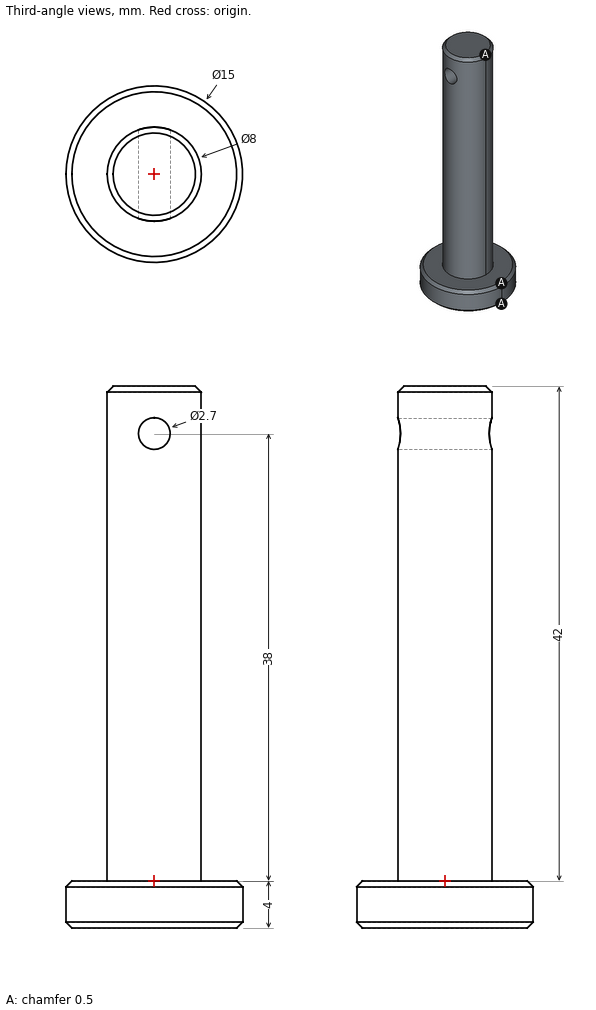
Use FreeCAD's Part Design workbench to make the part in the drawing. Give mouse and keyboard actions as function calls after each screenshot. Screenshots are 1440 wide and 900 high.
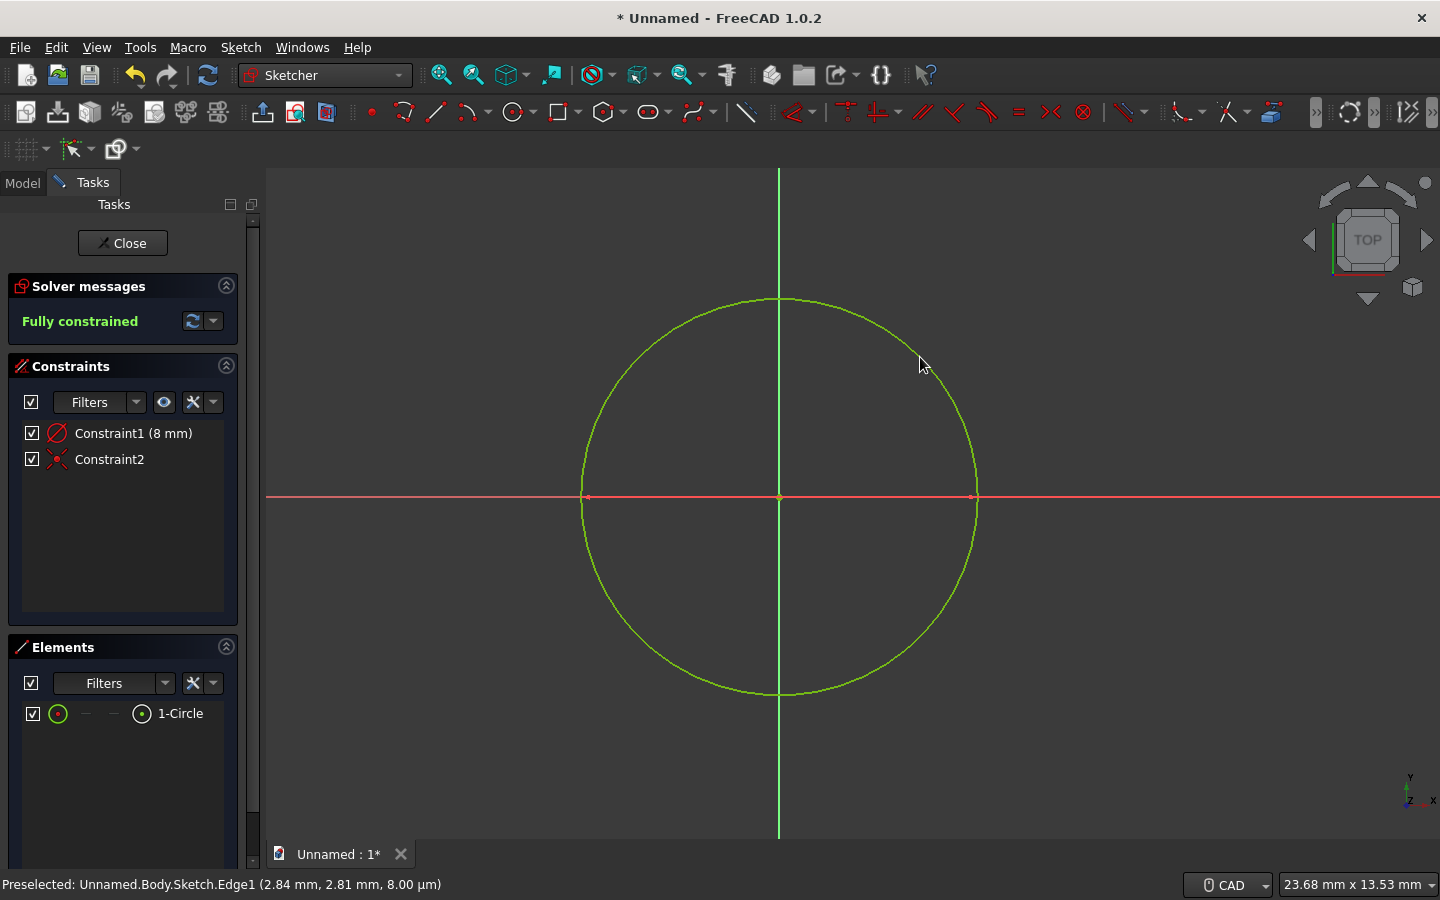
click(123, 243)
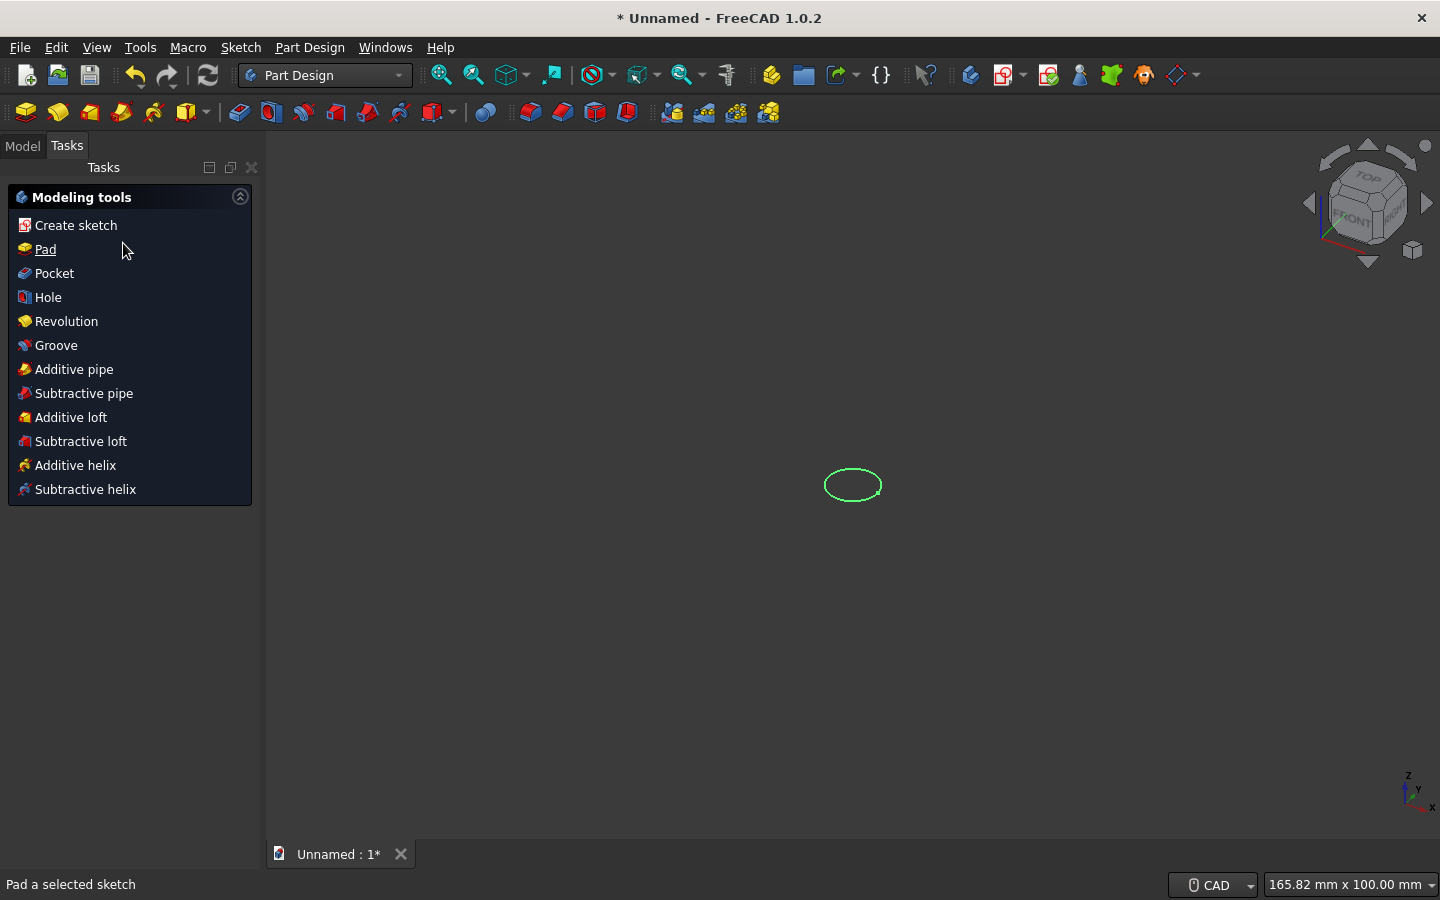
click(26, 112)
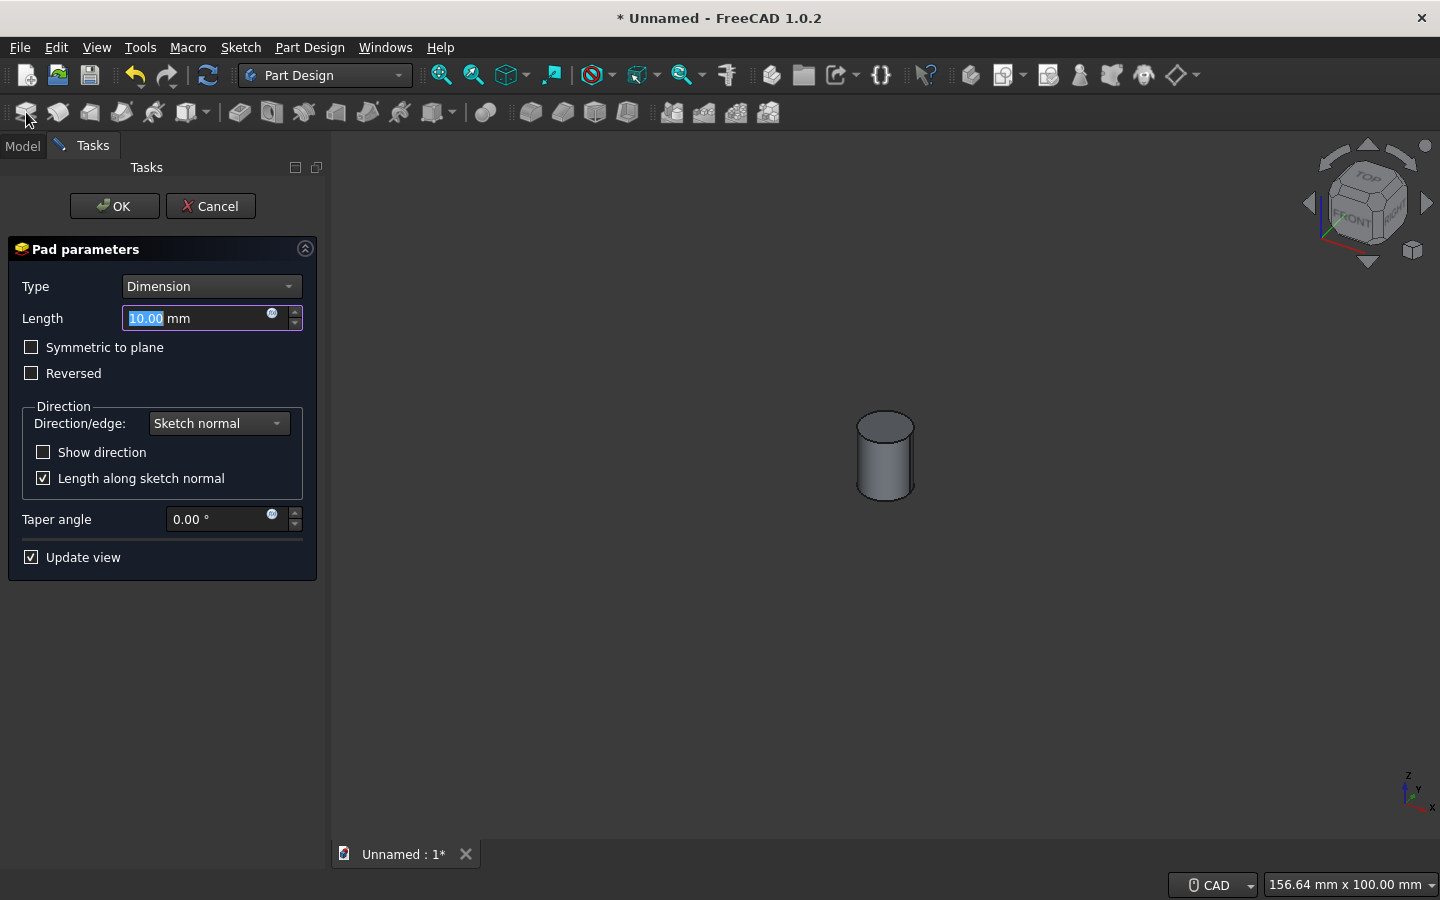
text(42)
key(Tab)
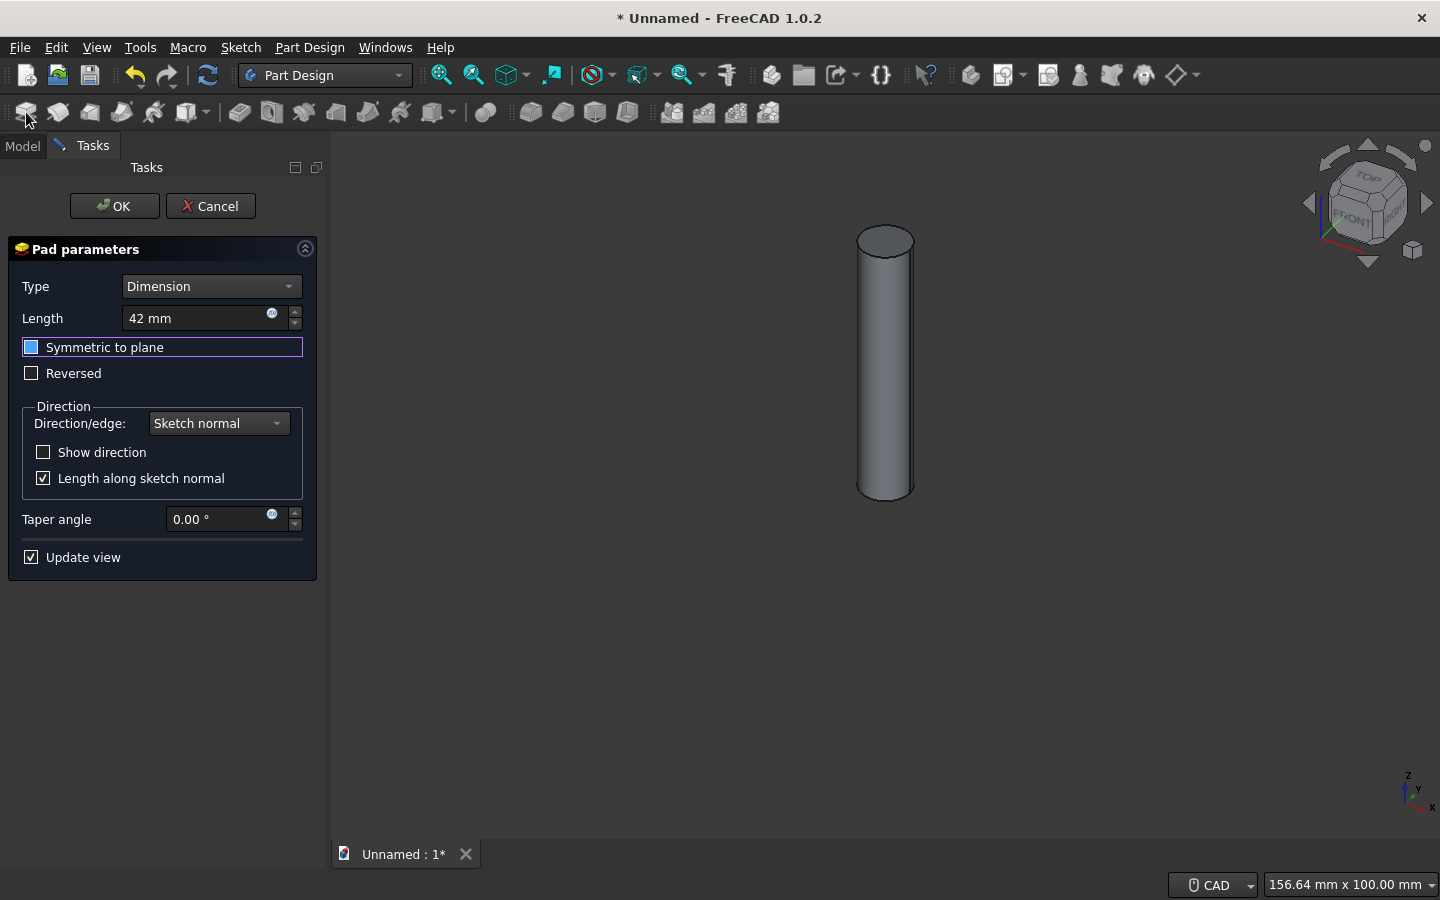
click(115, 206)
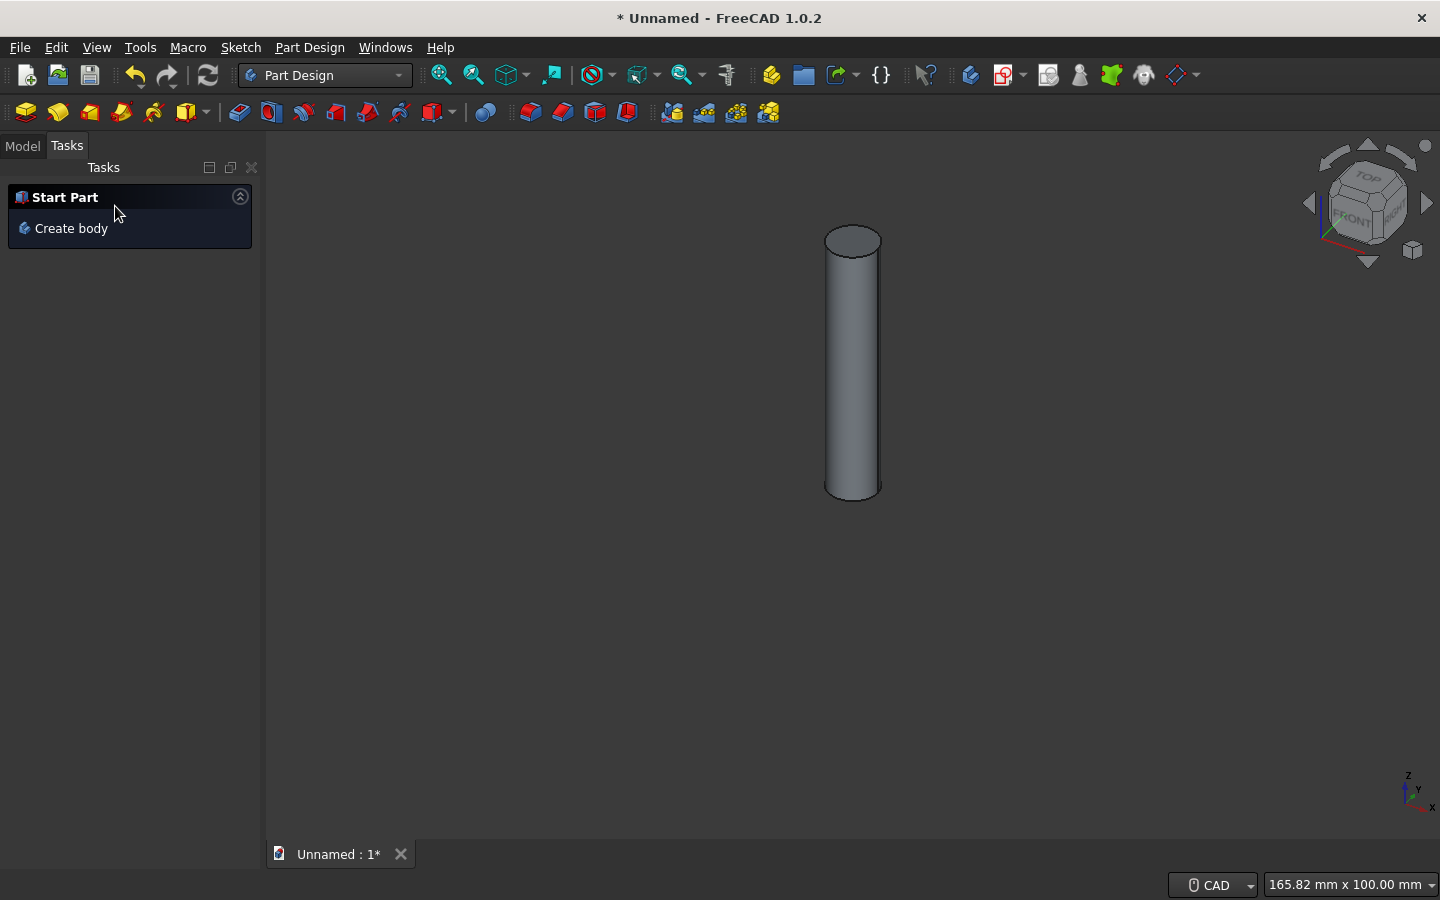
key(v)
key(f)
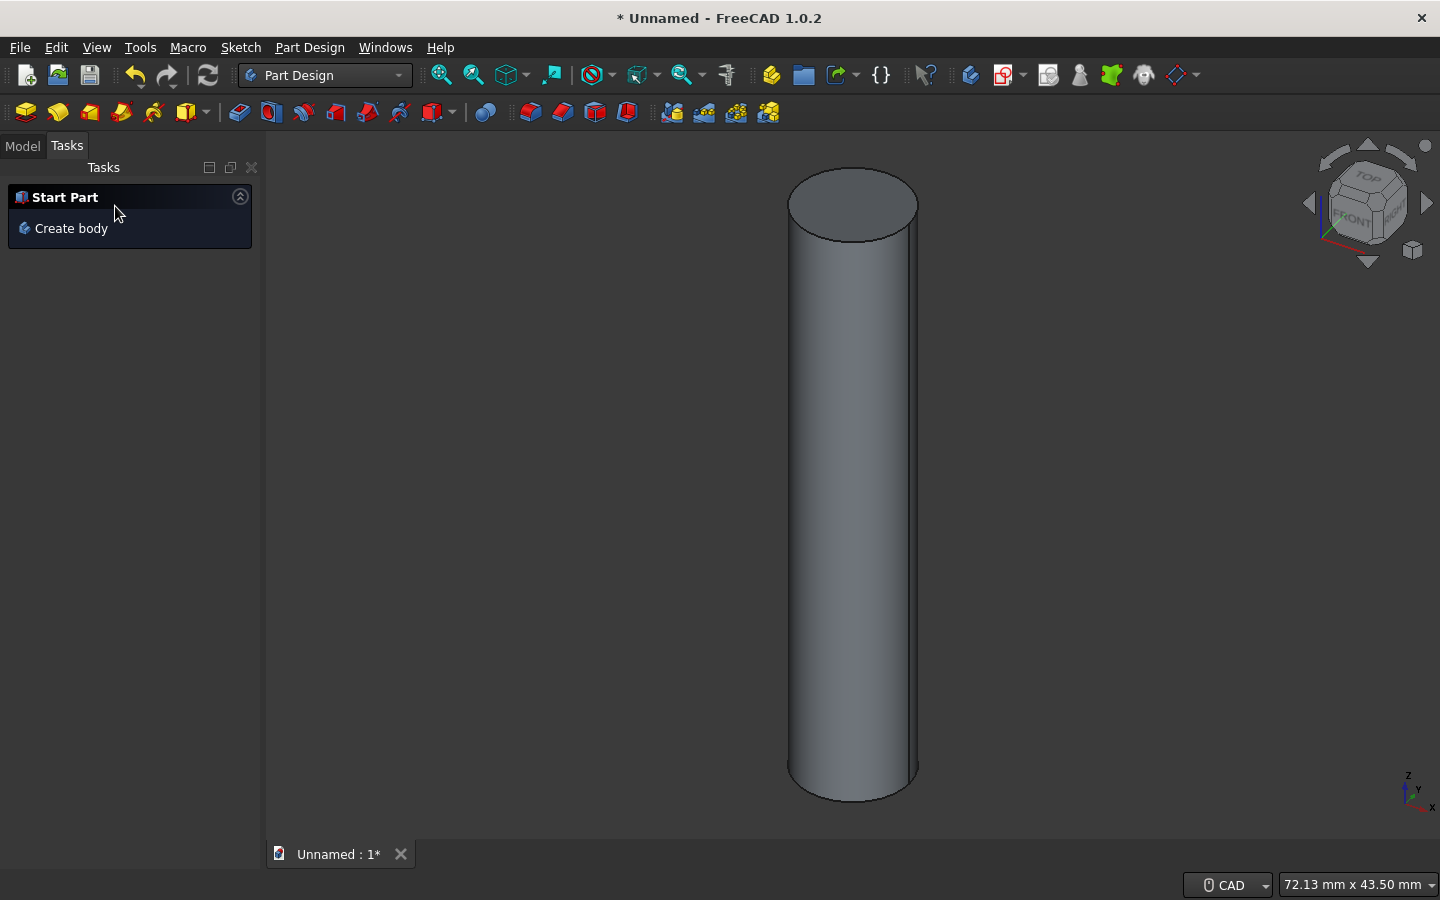
key(5)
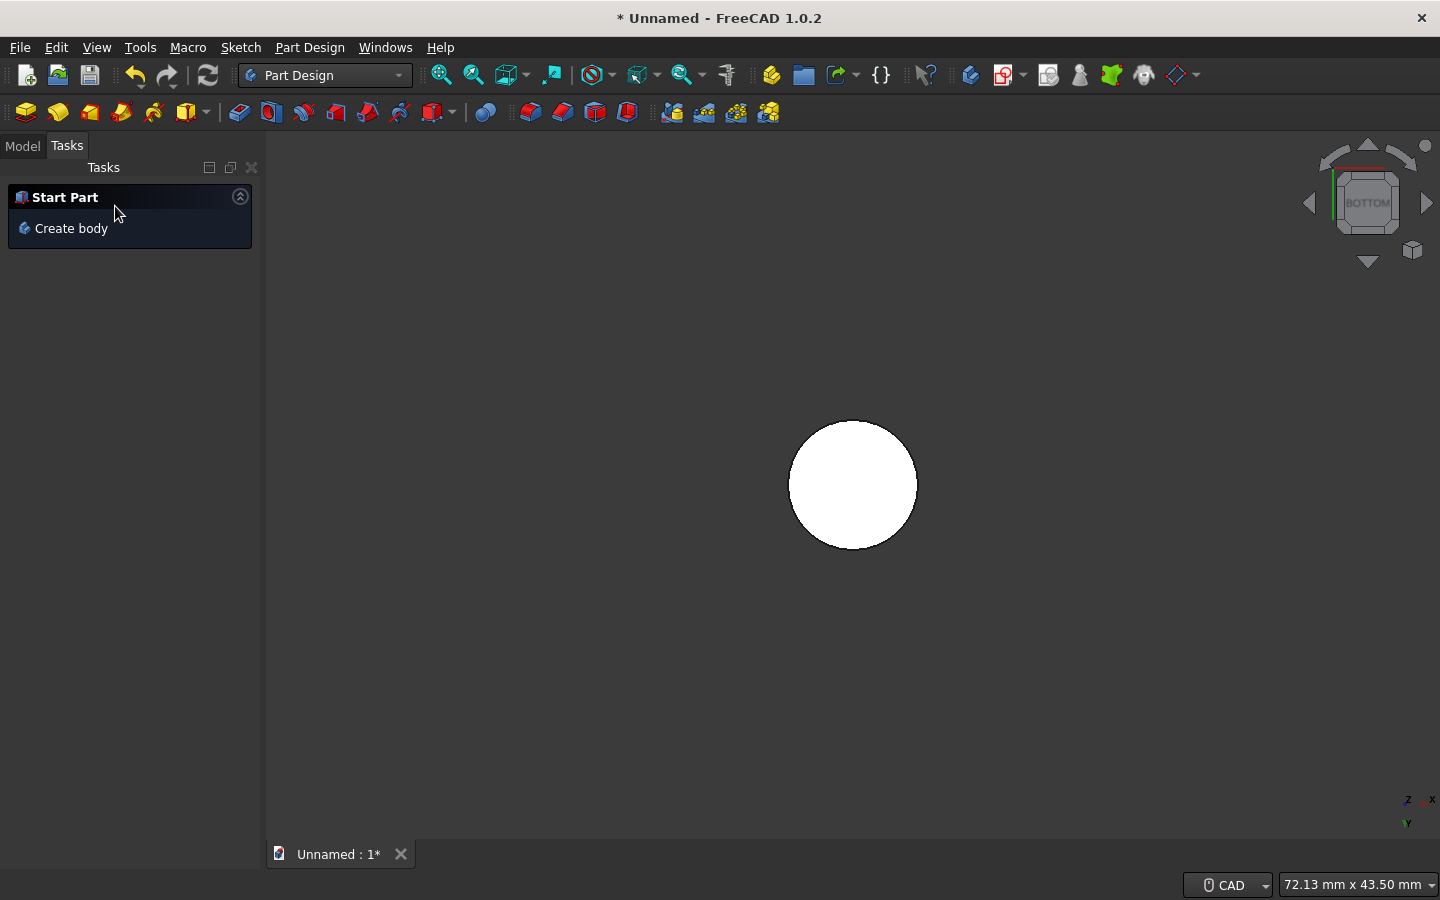
click(442, 76)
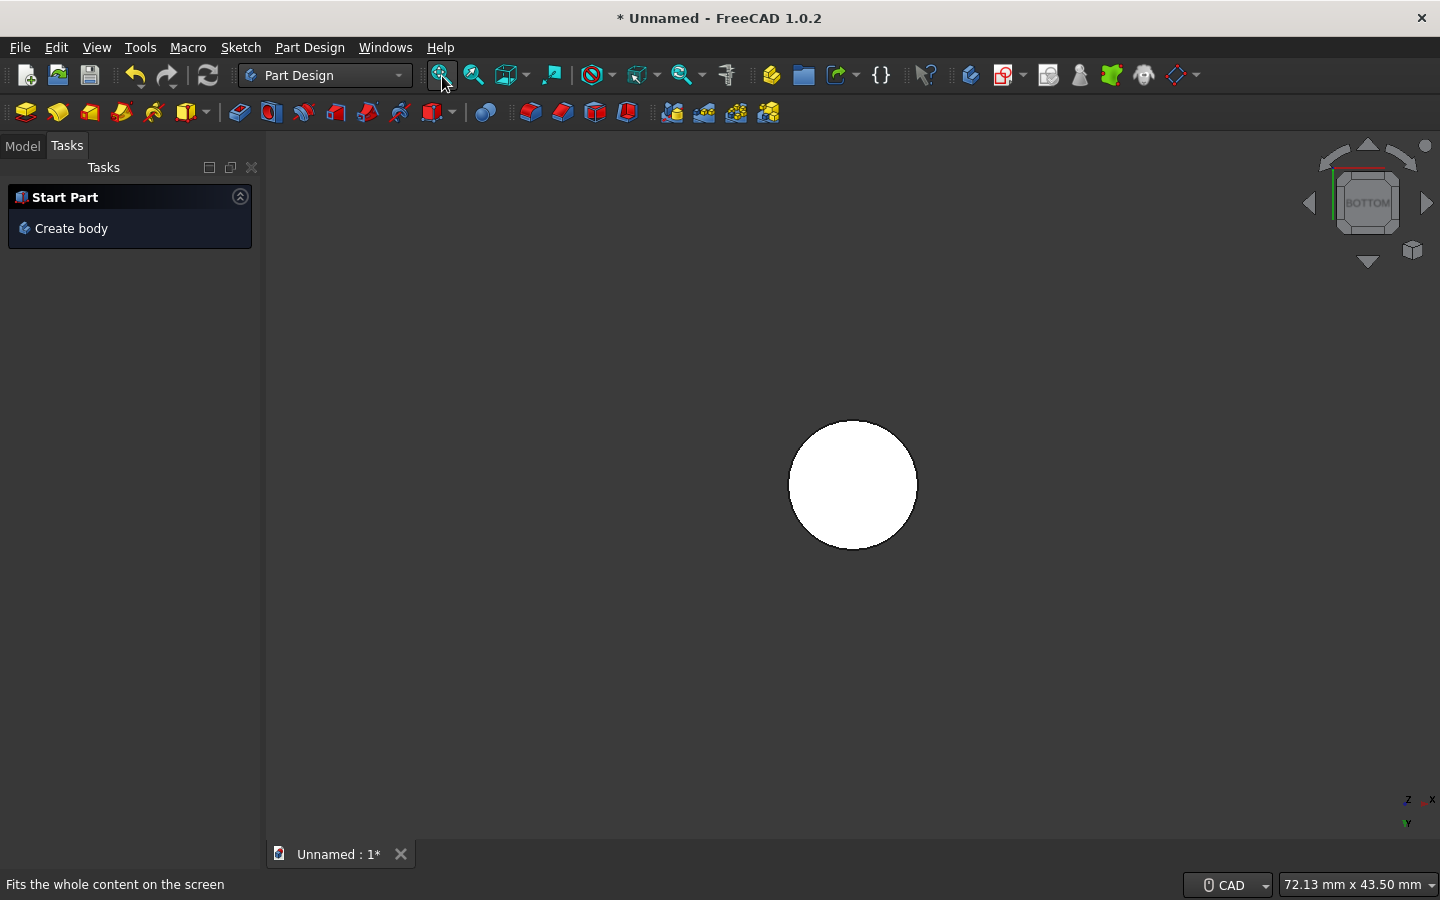
click(853, 484)